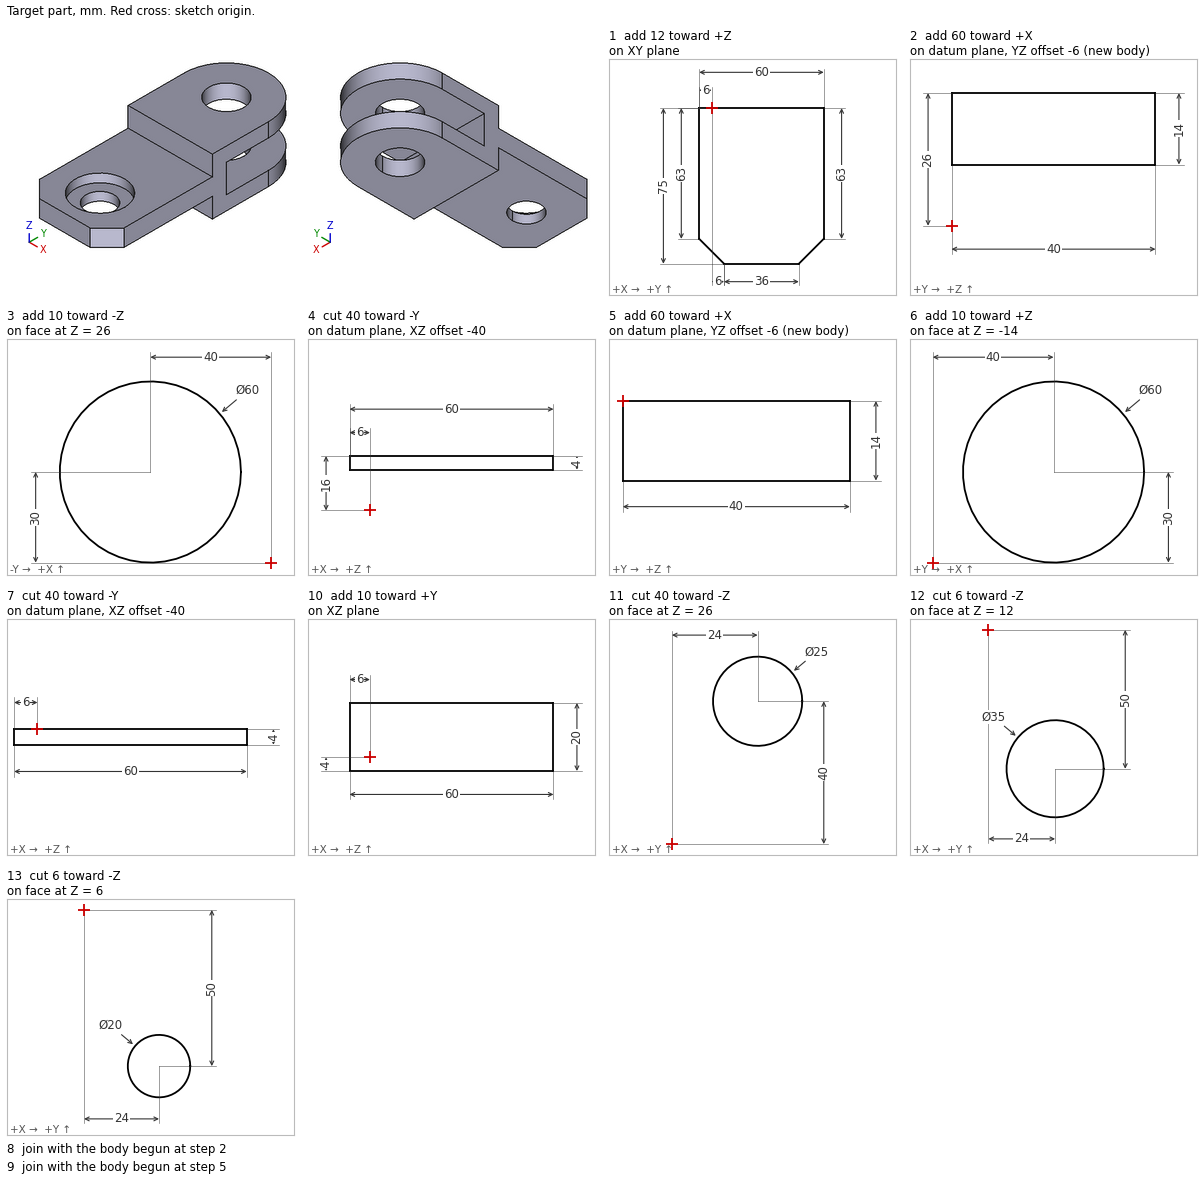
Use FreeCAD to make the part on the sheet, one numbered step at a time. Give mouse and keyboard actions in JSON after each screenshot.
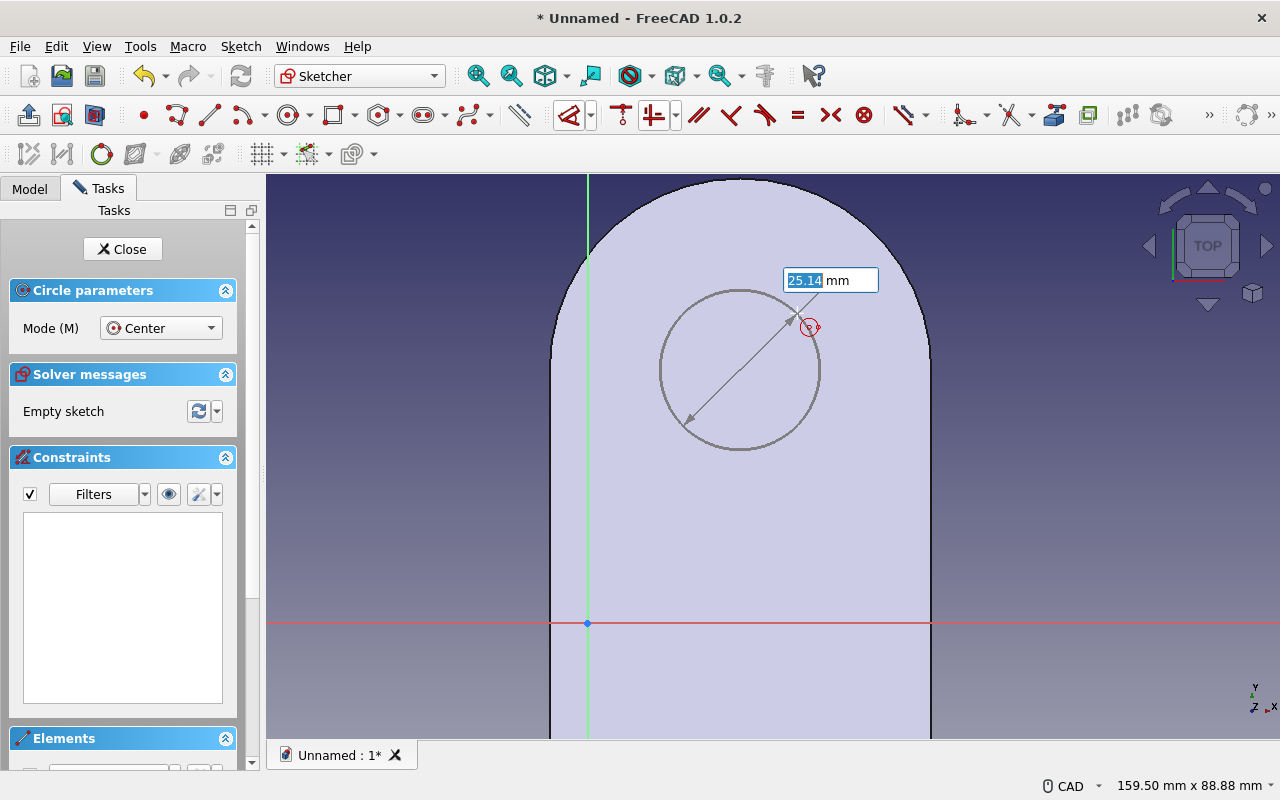
{"action": "type", "text": "25"}
{"action": "key", "text": "Return"}
{"action": "key", "text": "Escape"}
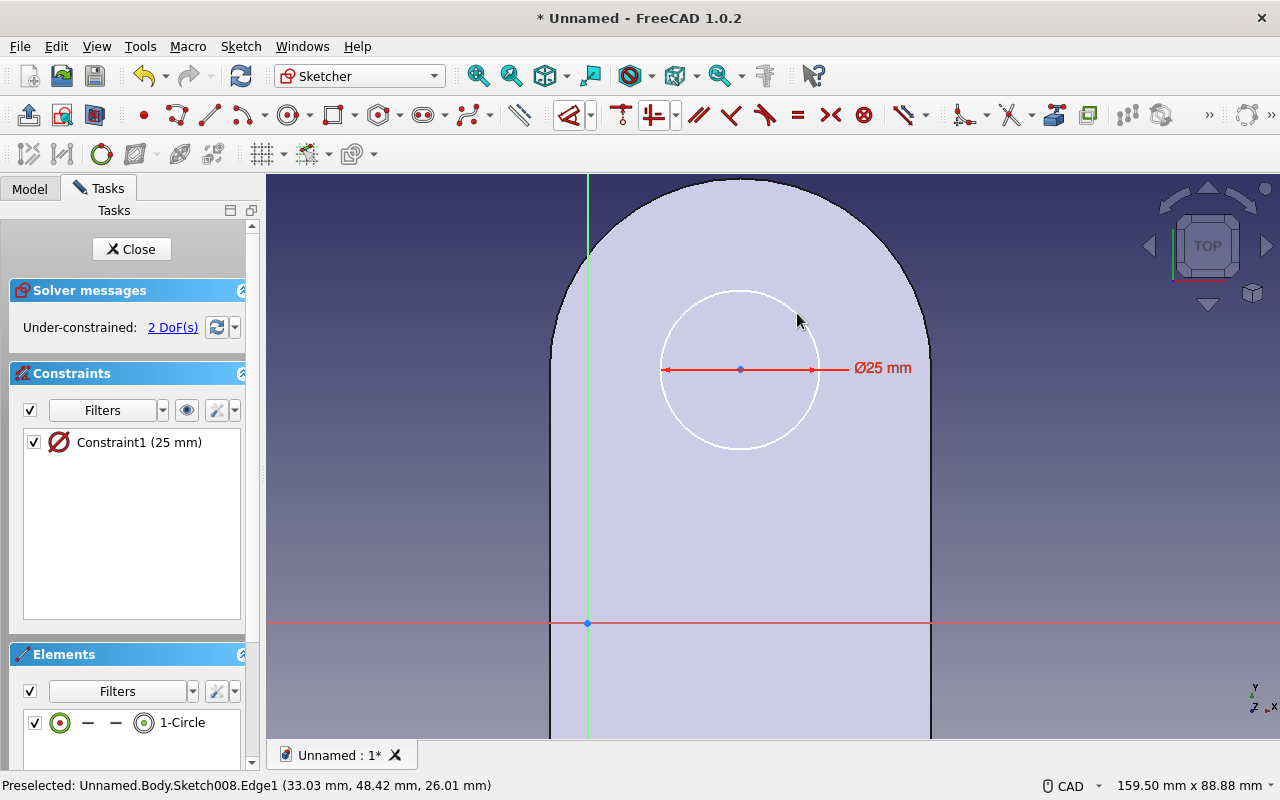
{"action": "left_click", "coordinate": [740, 370]}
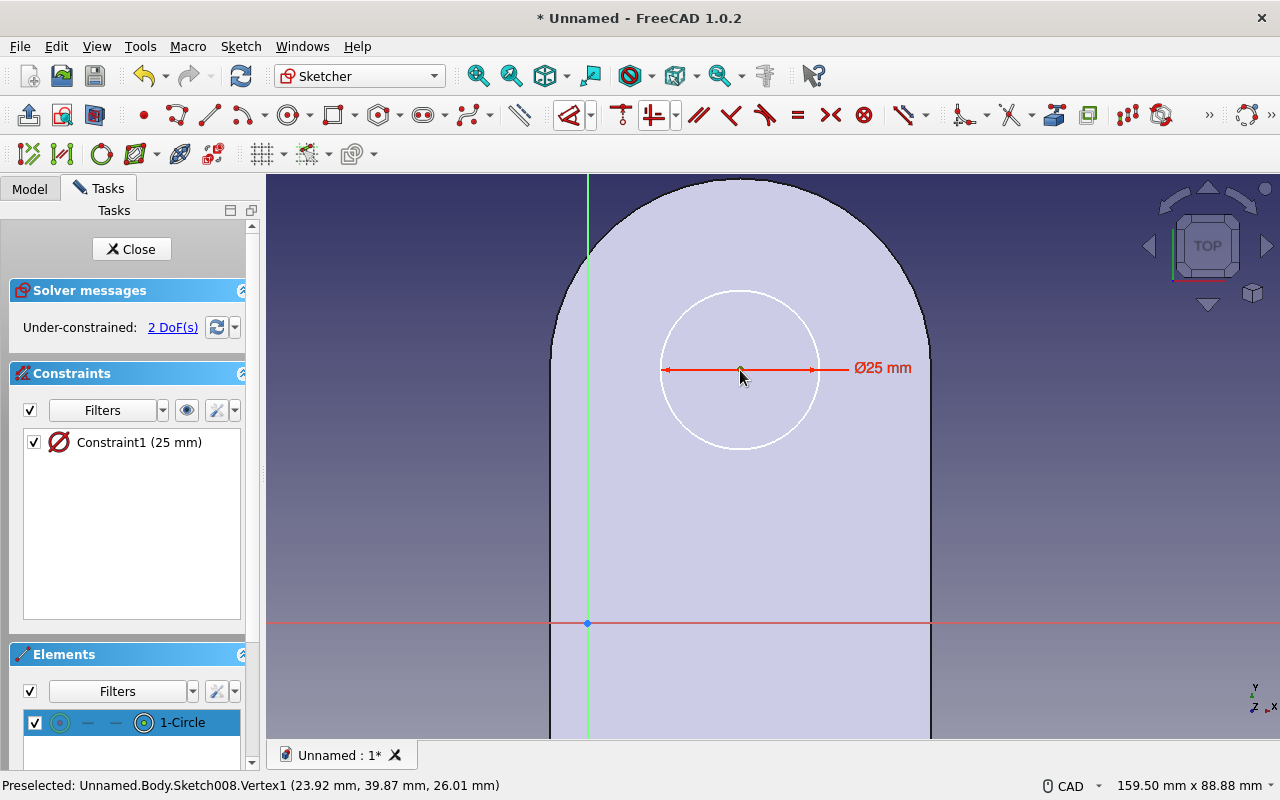
{"action": "key", "text": "l"}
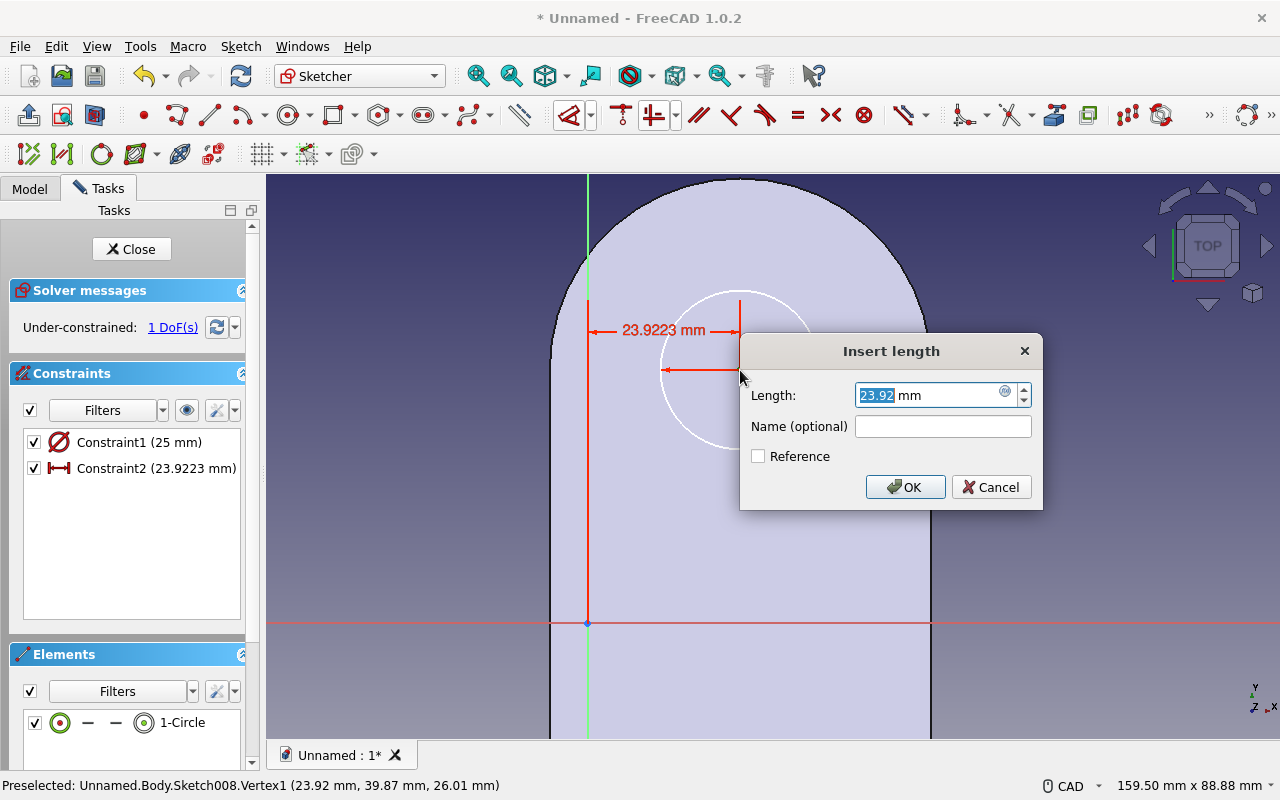
{"action": "type", "text": "24"}
{"action": "key", "text": "Return"}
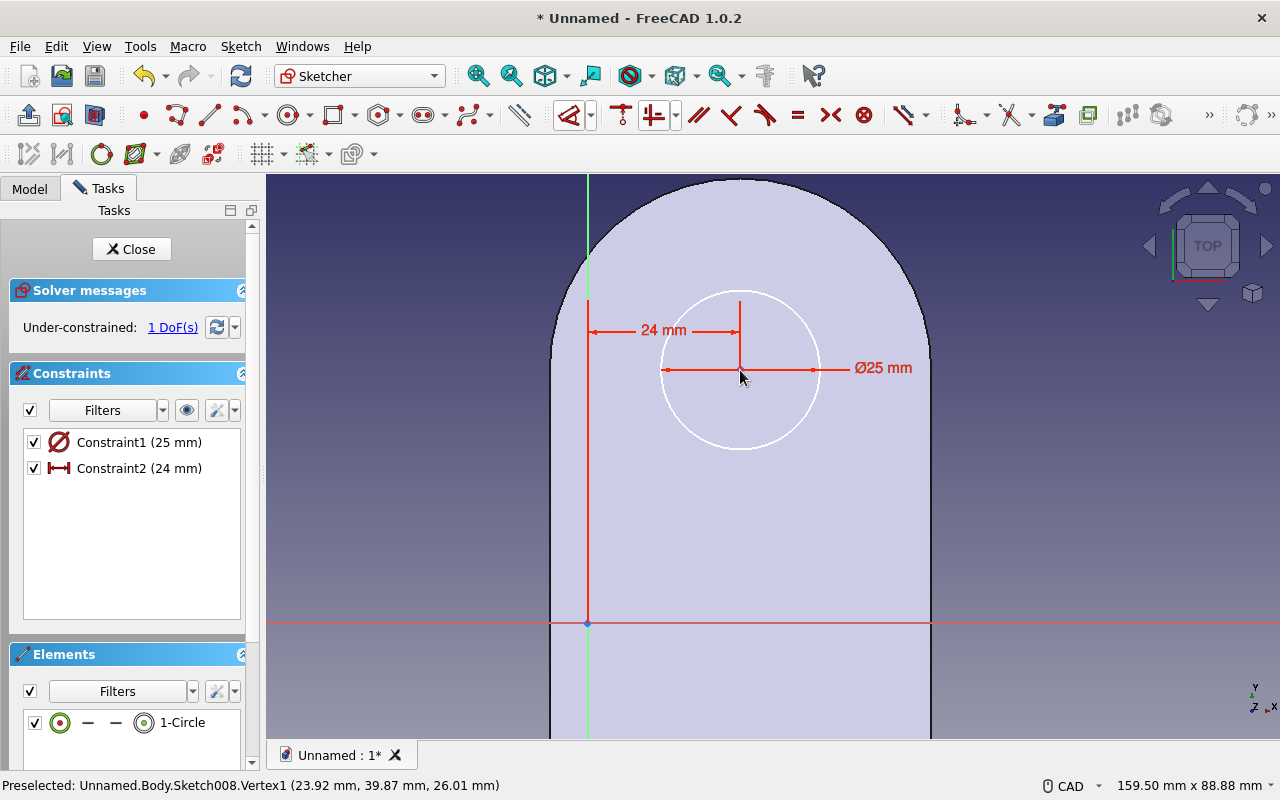
{"action": "left_click", "coordinate": [740, 370]}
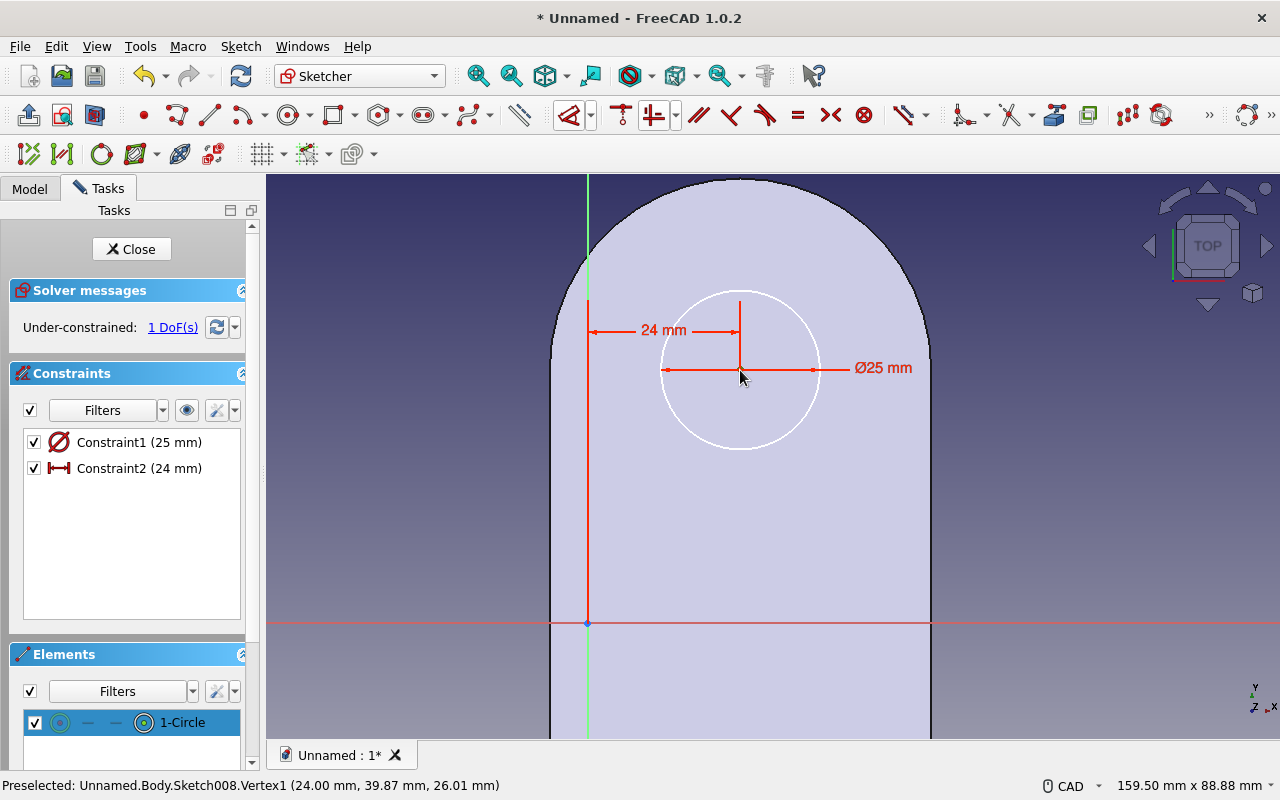
{"action": "key", "text": "i"}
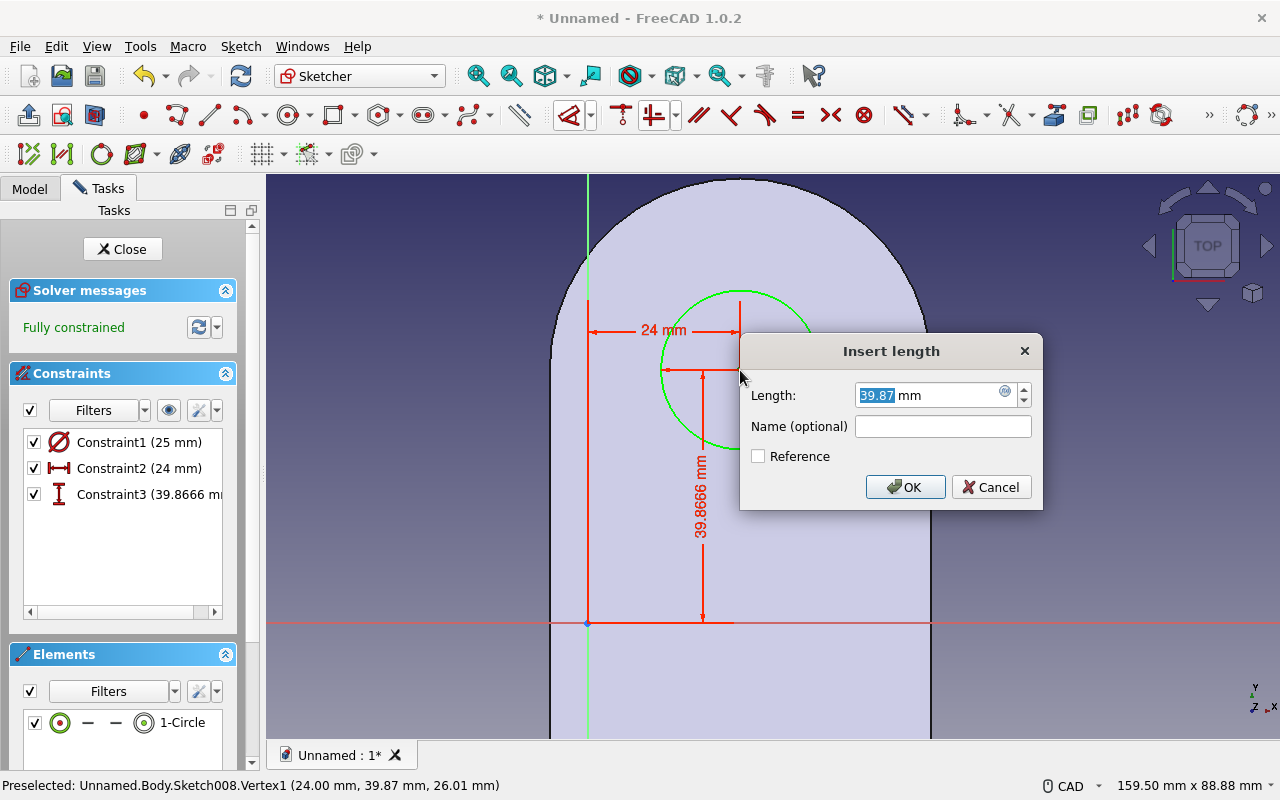
{"action": "type", "text": "40"}
{"action": "key", "text": "Return"}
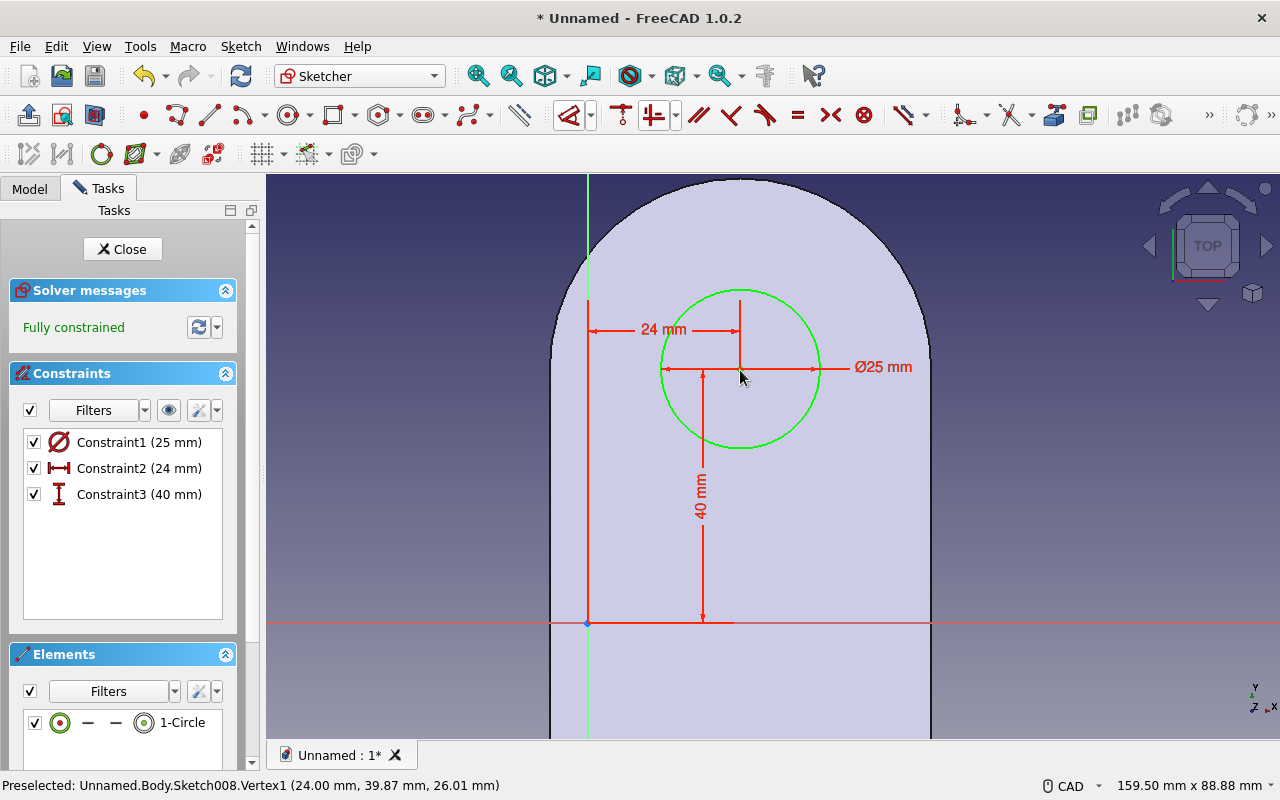
{"action": "left_click", "coordinate": [123, 249]}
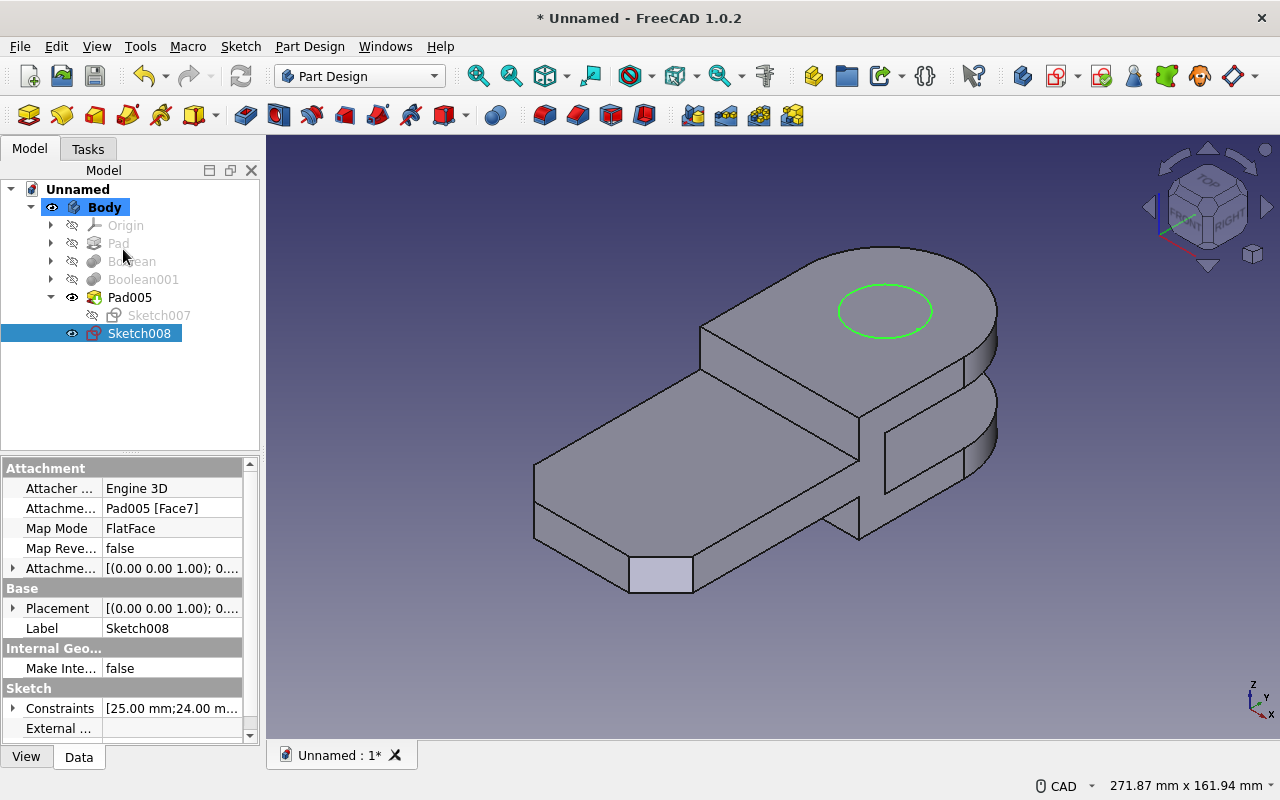
{"action": "left_click", "coordinate": [246, 116]}